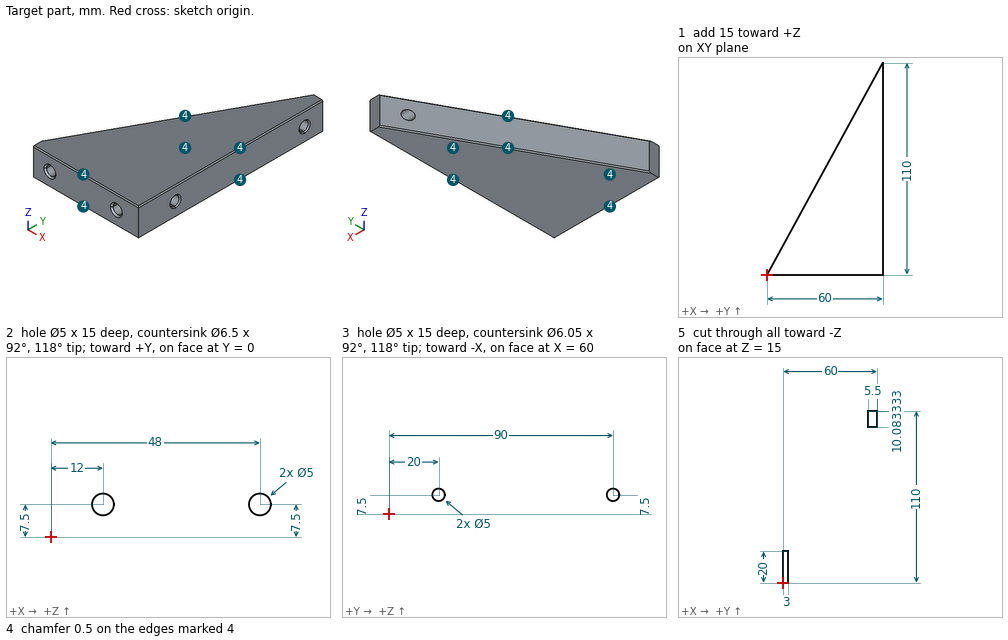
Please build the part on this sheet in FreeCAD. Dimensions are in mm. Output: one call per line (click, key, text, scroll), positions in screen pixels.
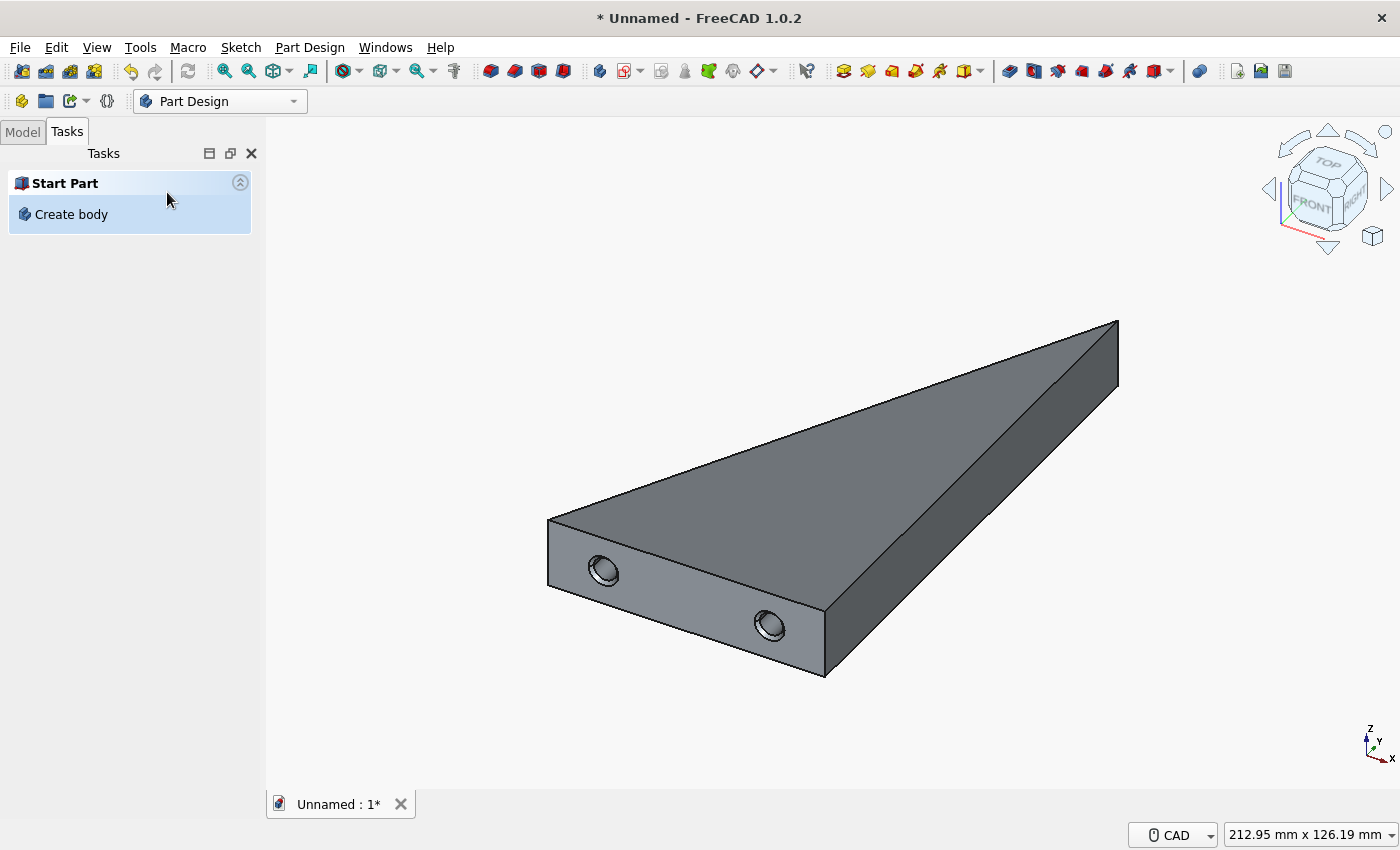
click(1097, 373)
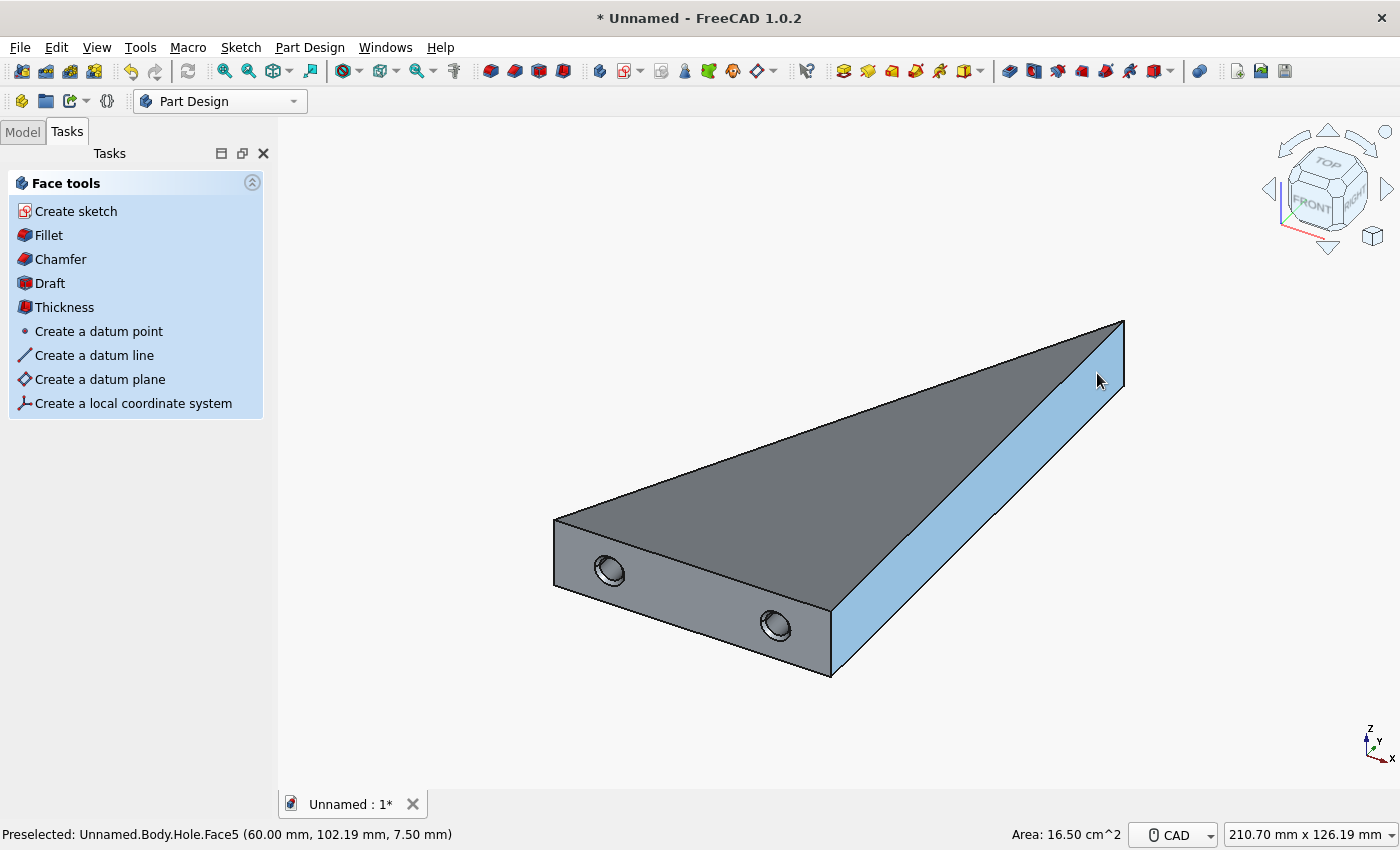
click(624, 72)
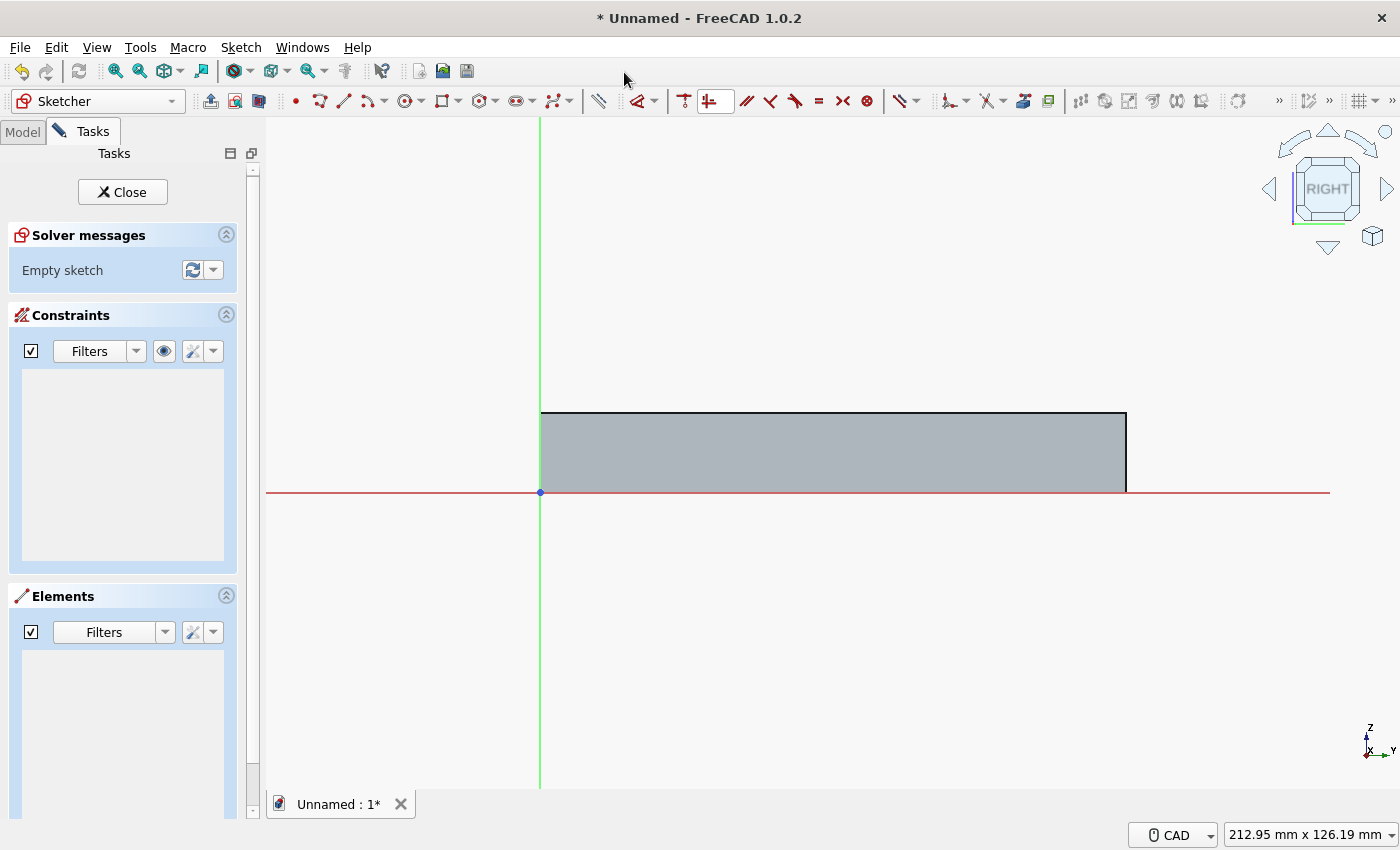
click(406, 102)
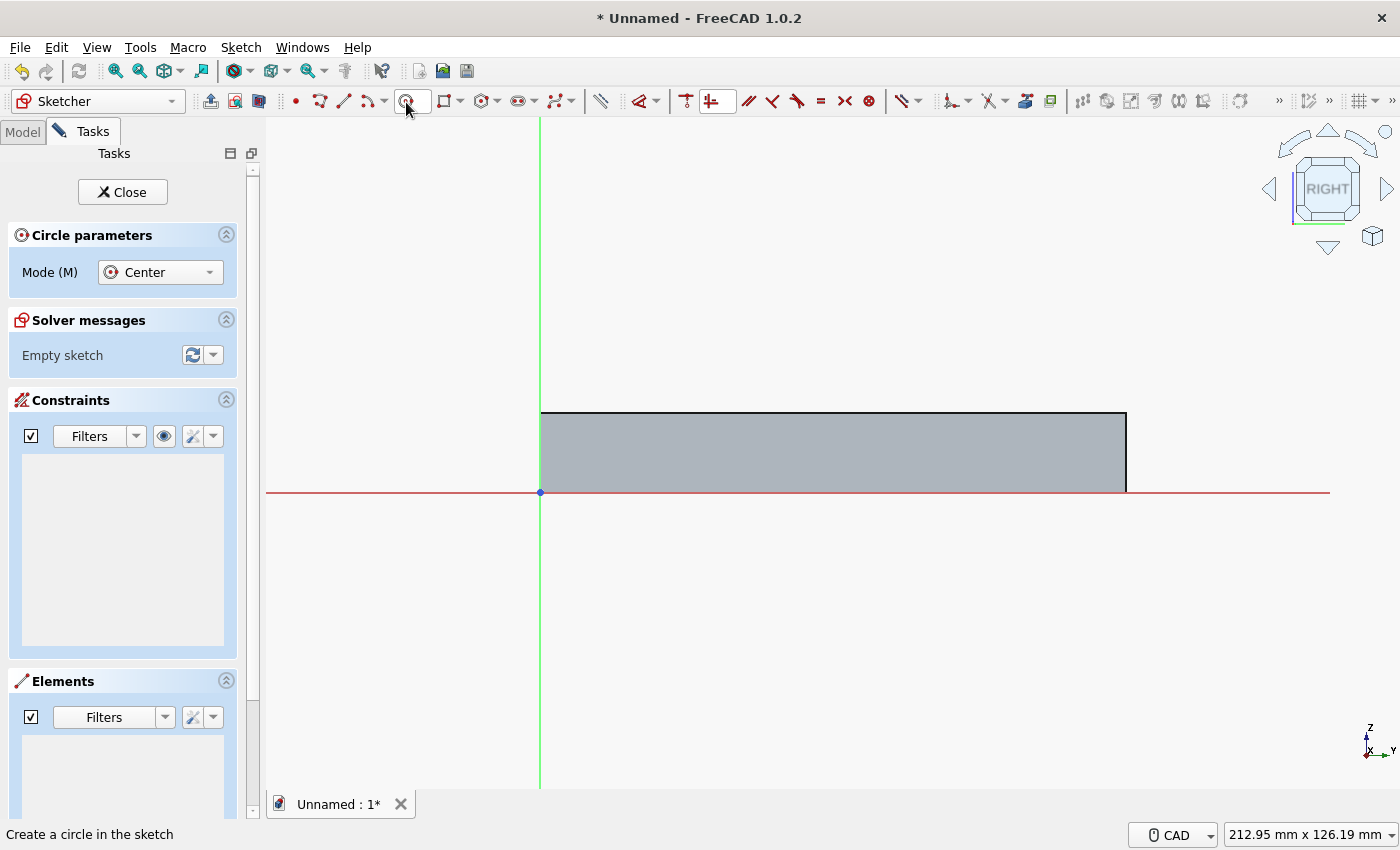
scroll(647, 453, up, 3)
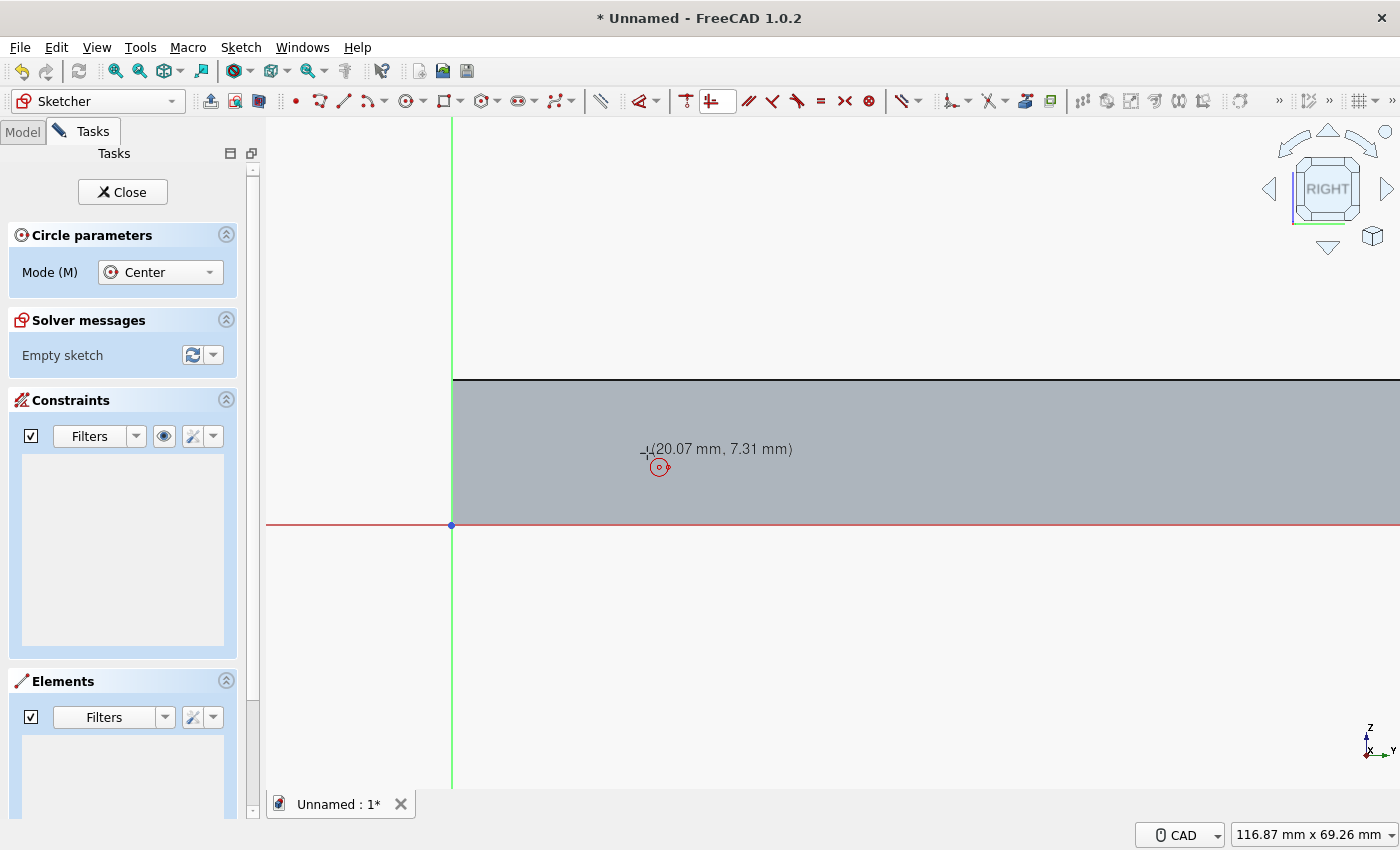
click(646, 453)
click(663, 435)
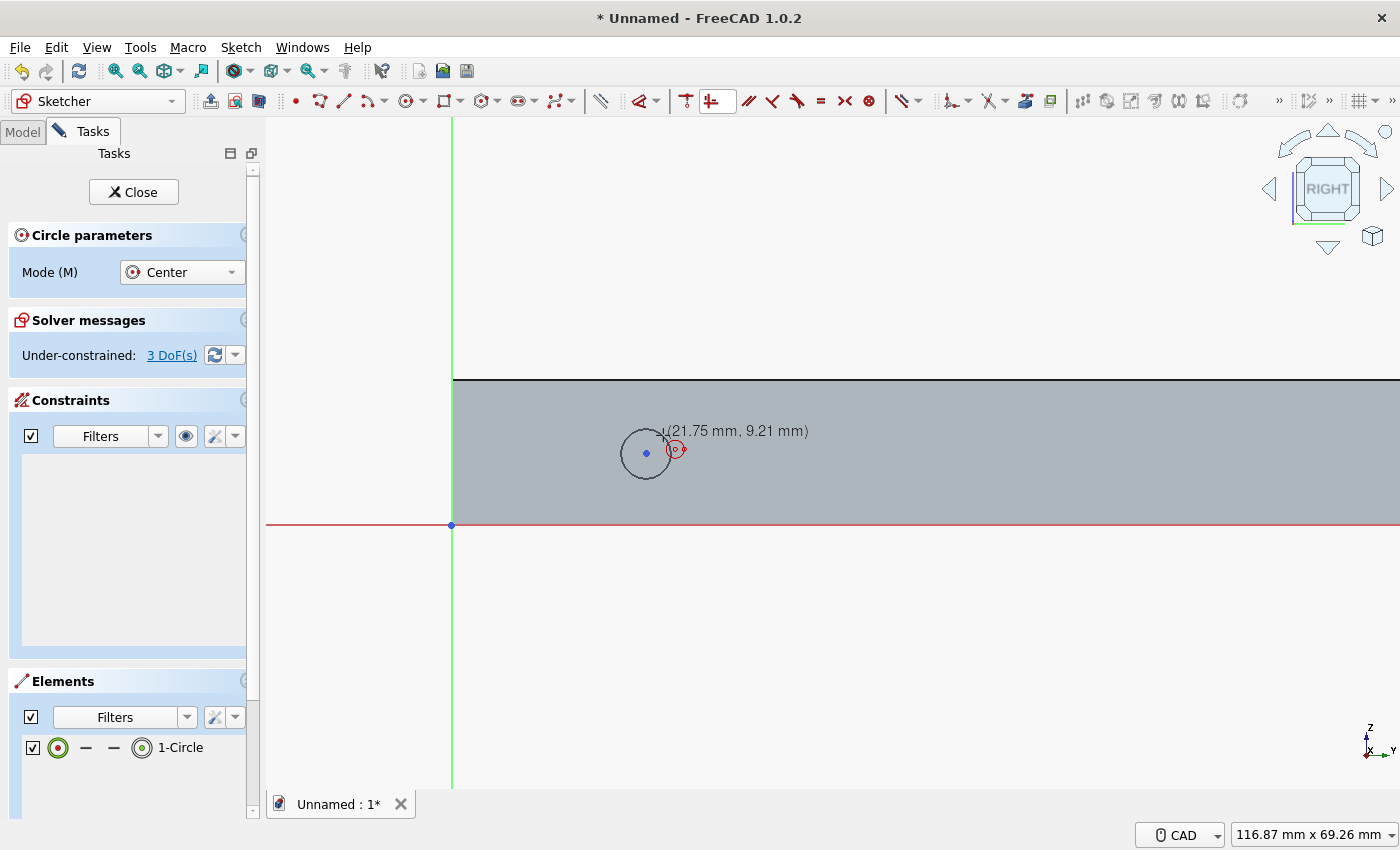
scroll(487, 405, down, 2)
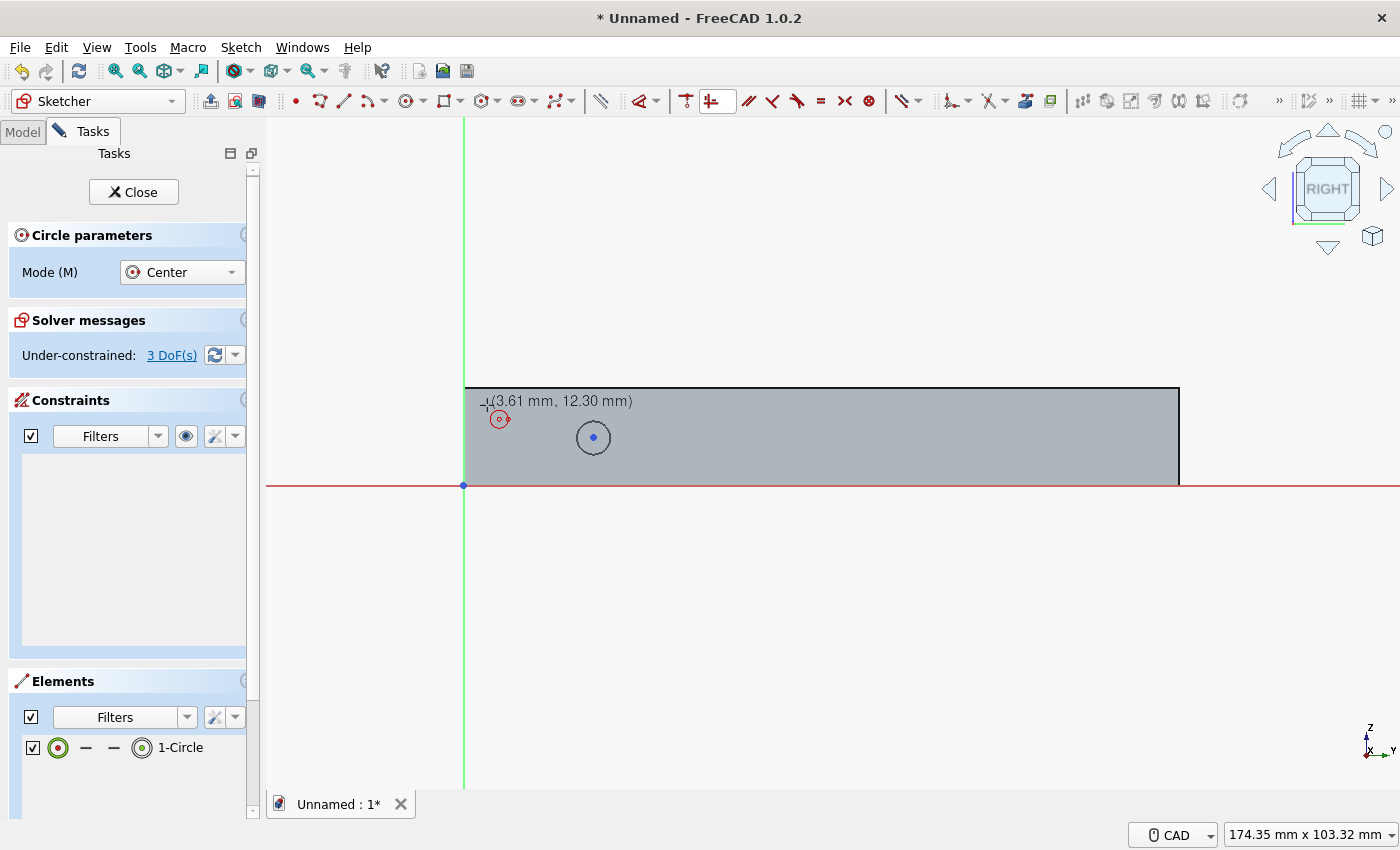
scroll(1049, 437, up, 2)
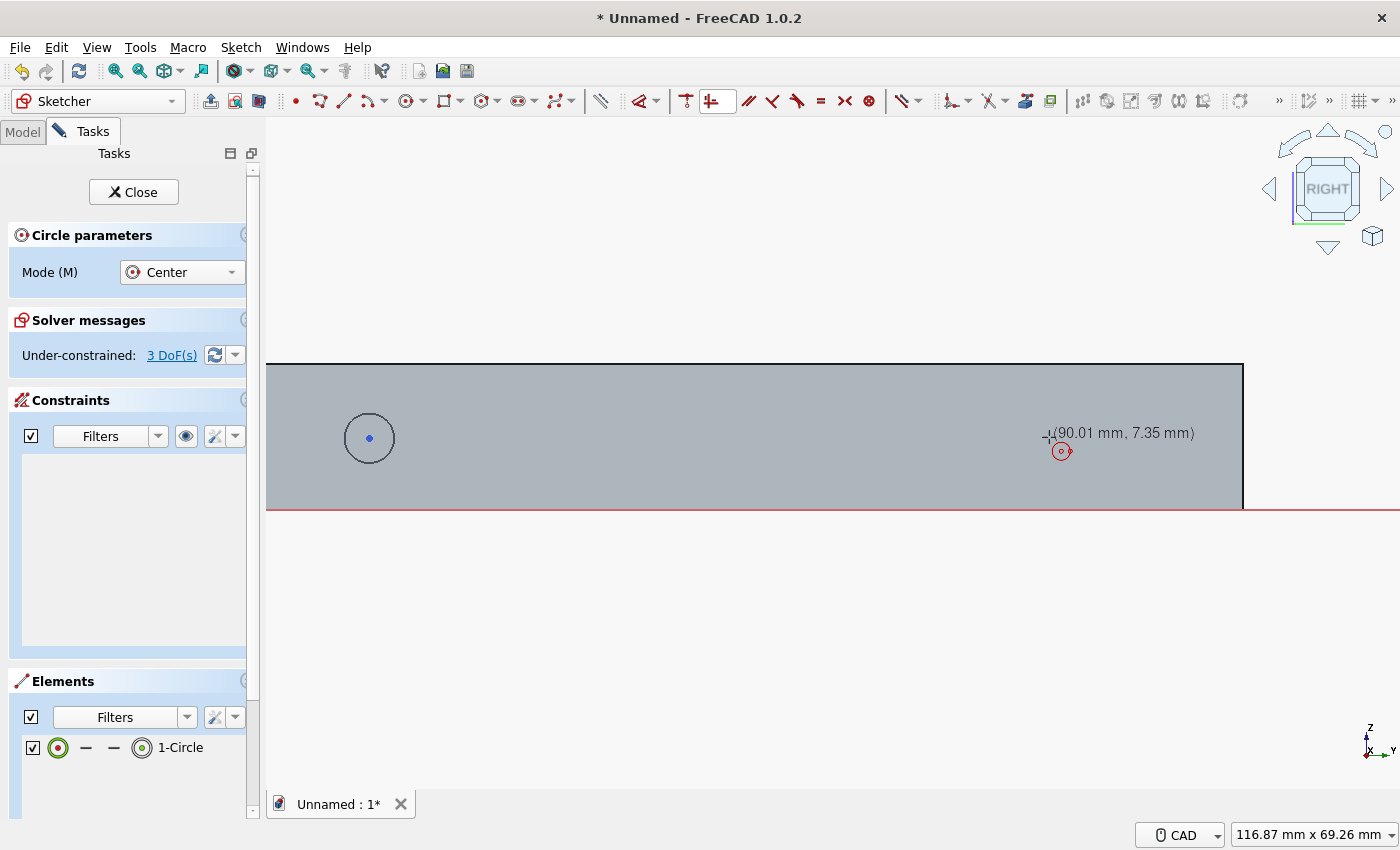
click(1049, 437)
click(1066, 420)
key(Escape)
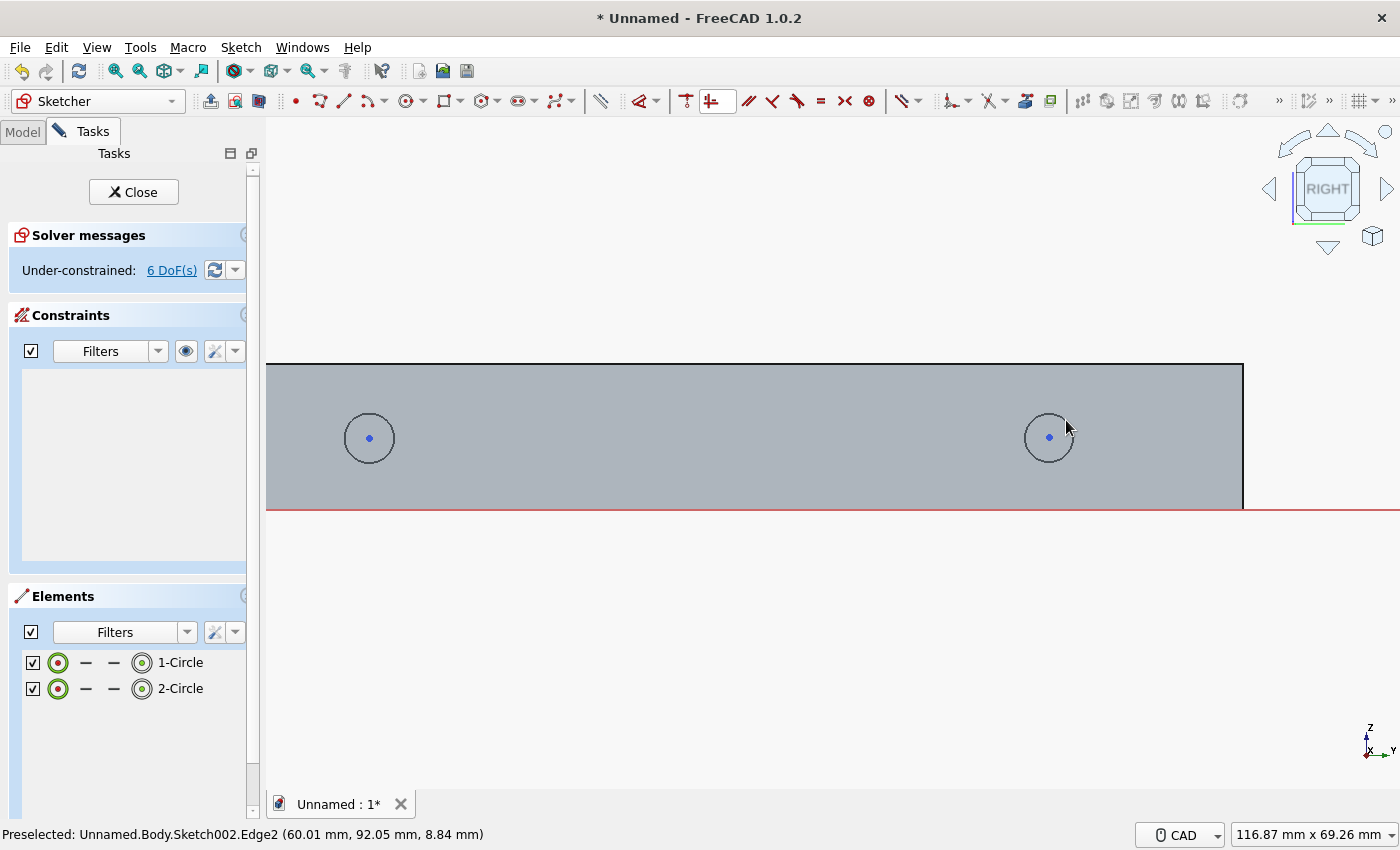
click(387, 421)